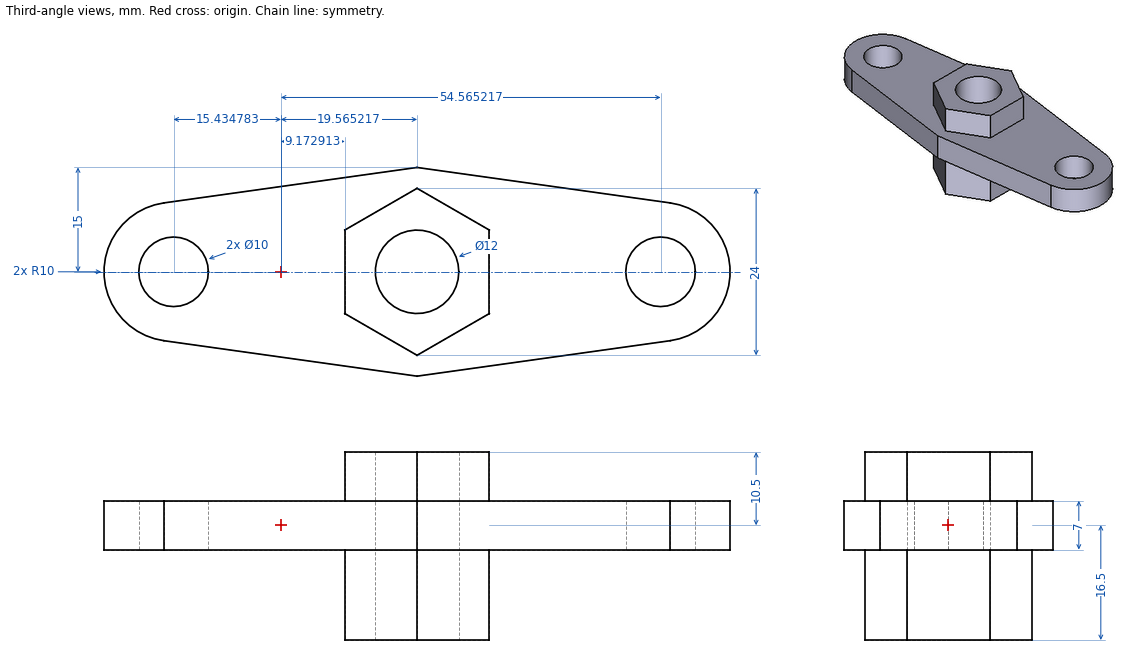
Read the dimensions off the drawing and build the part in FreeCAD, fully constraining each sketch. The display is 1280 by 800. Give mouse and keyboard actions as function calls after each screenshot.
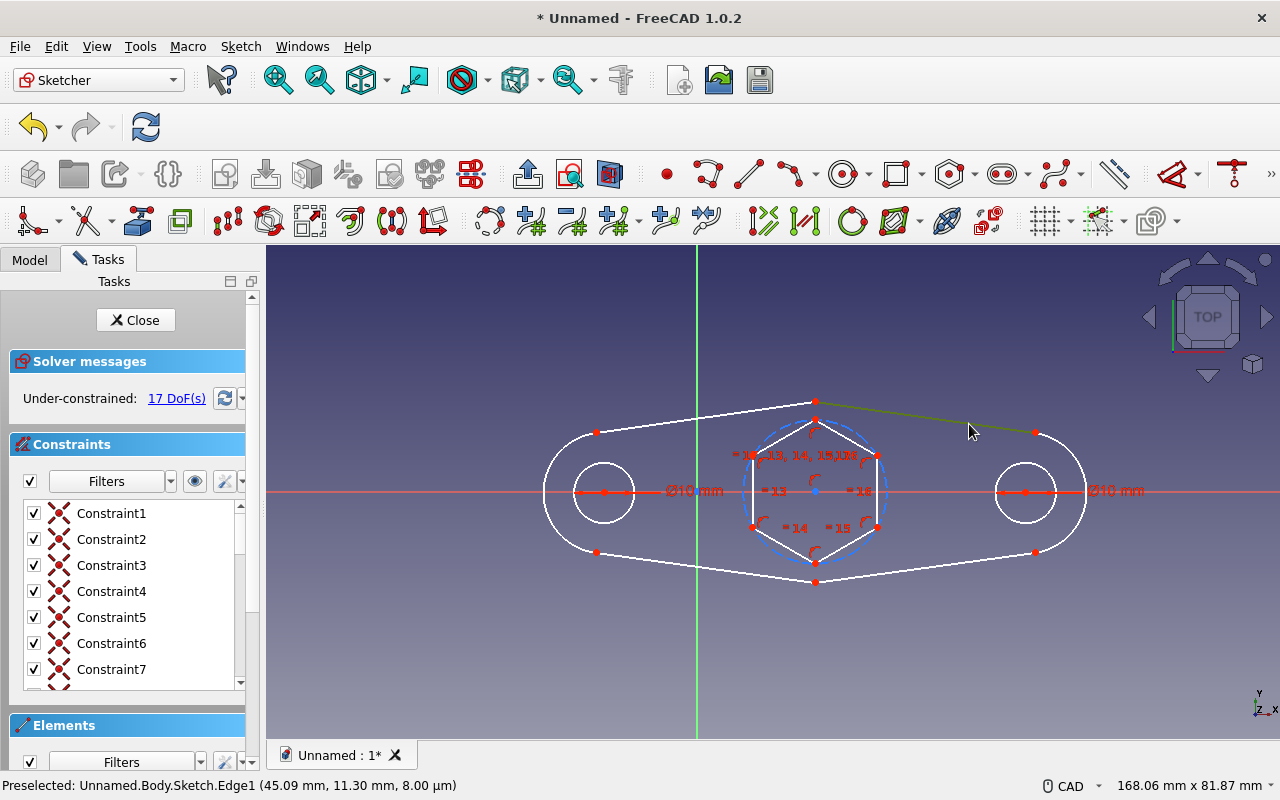
click(1077, 526)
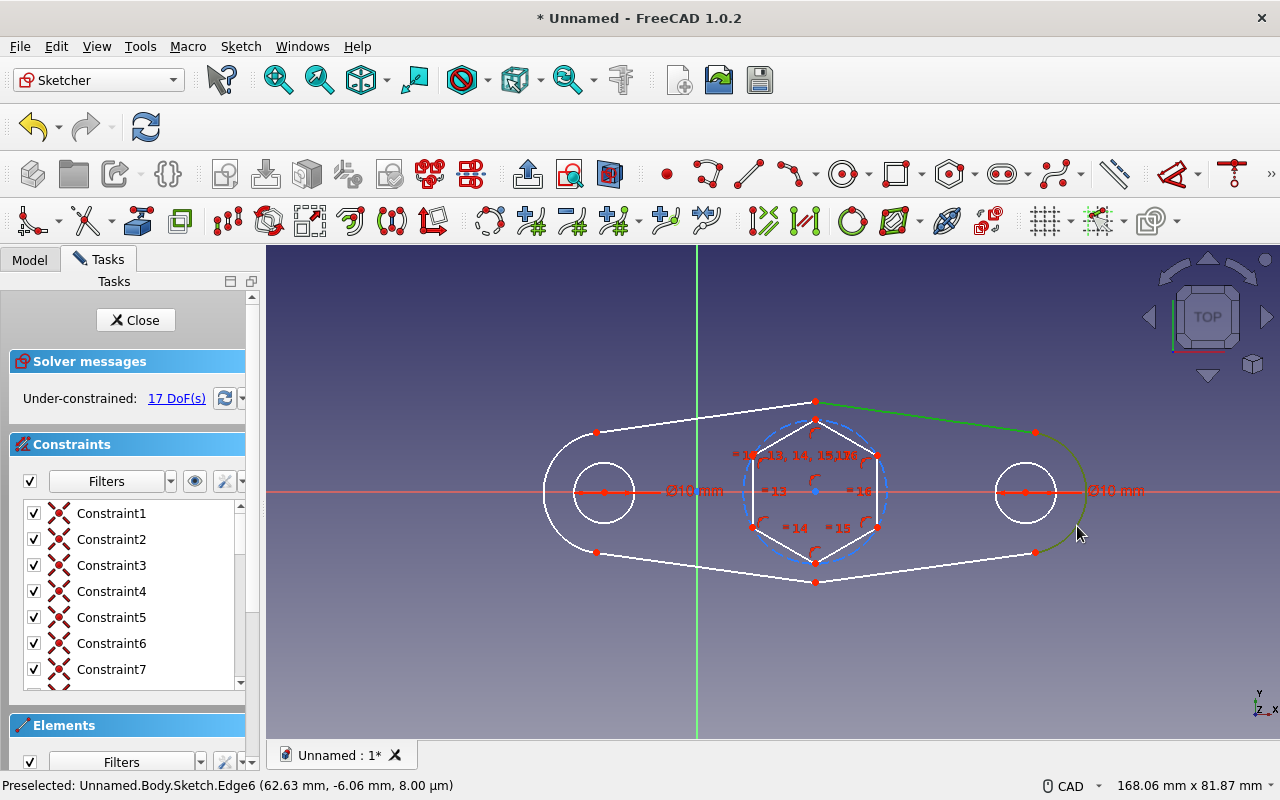
key(t)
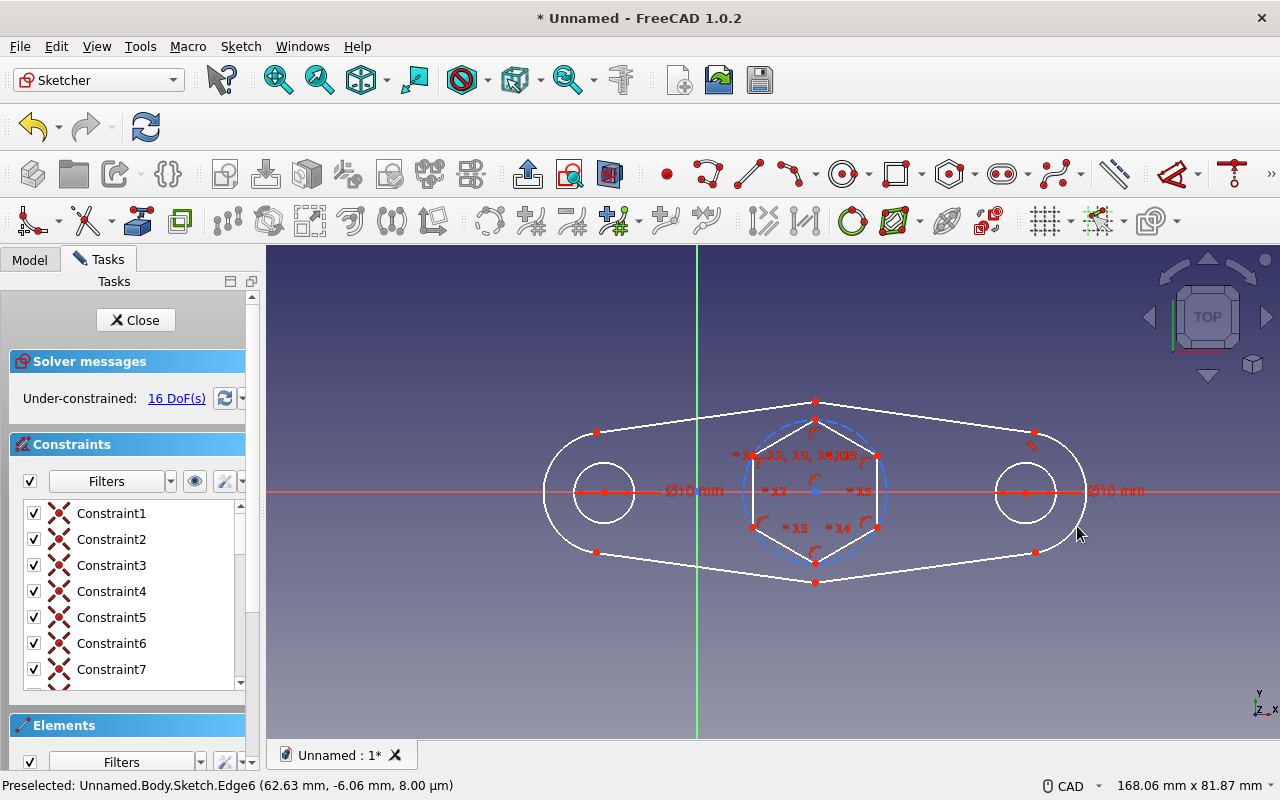
click(749, 411)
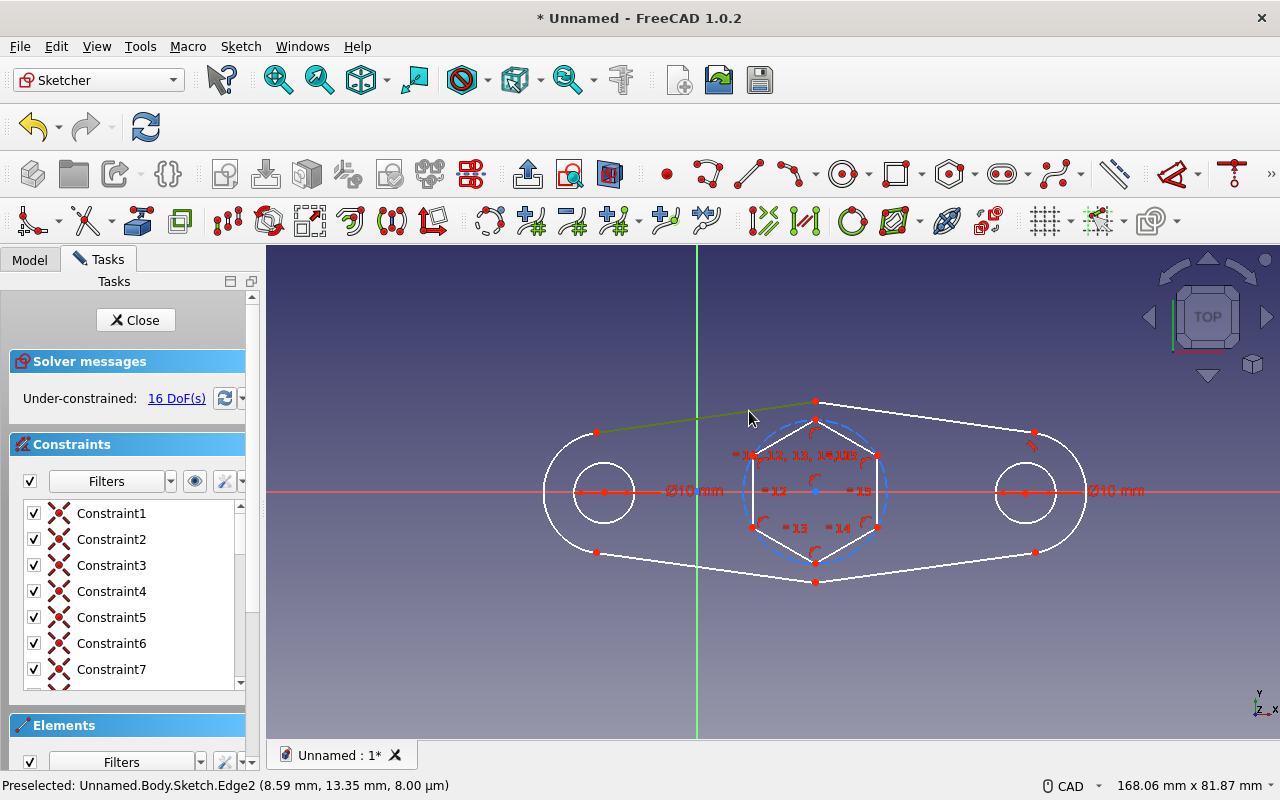
click(553, 460)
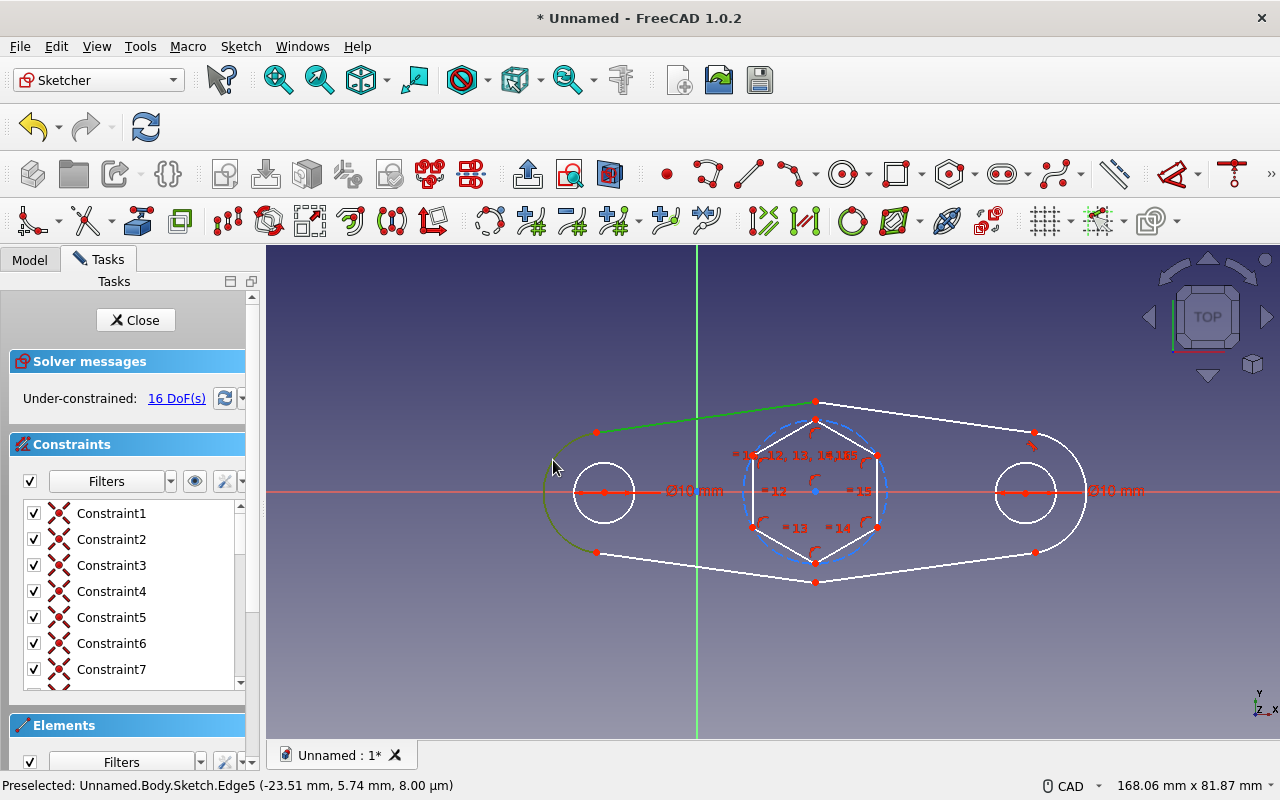
key(t)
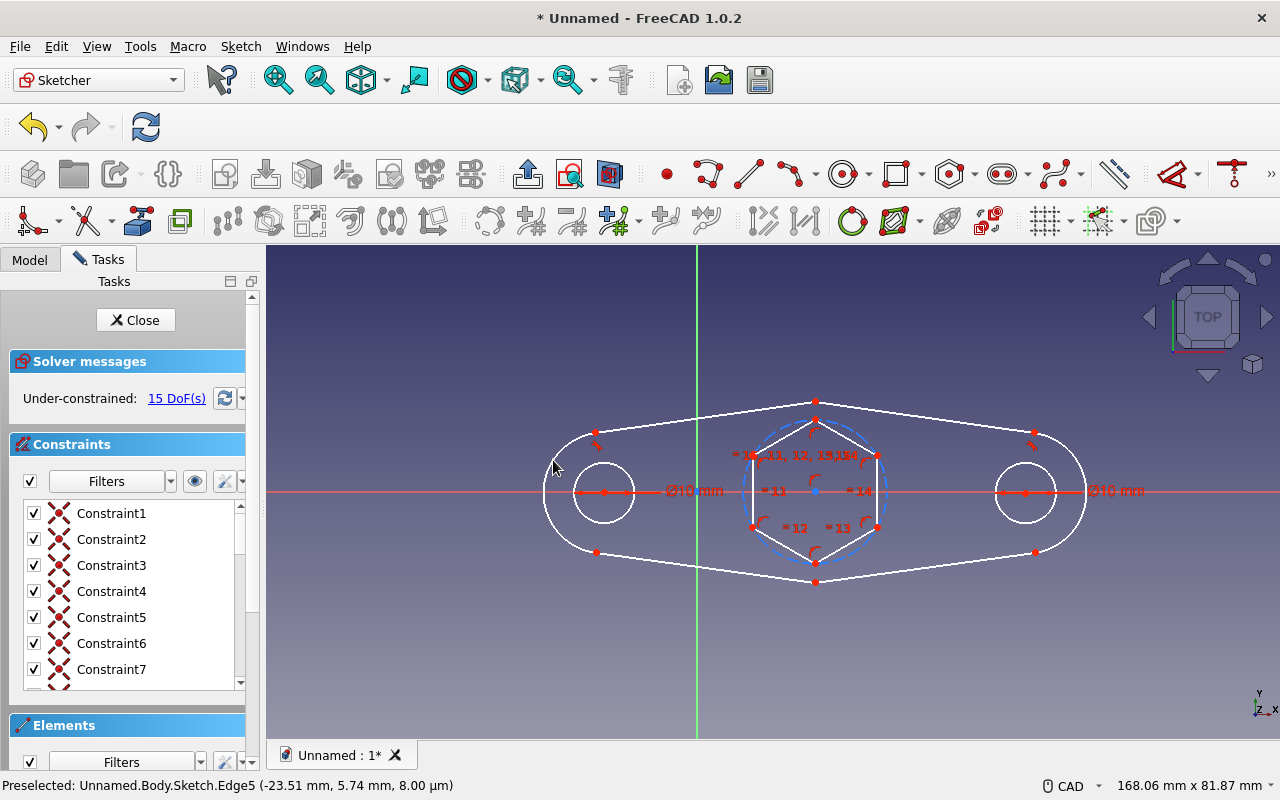
click(662, 562)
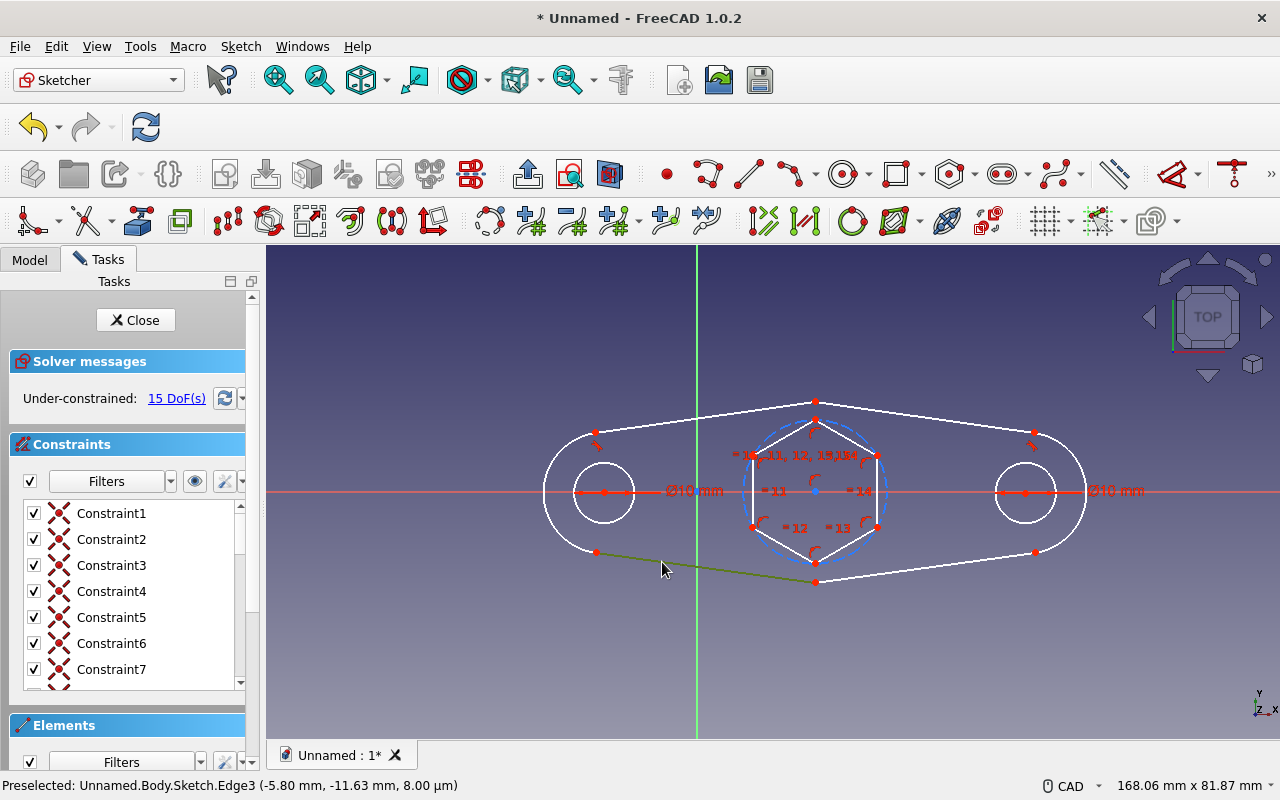
click(553, 460)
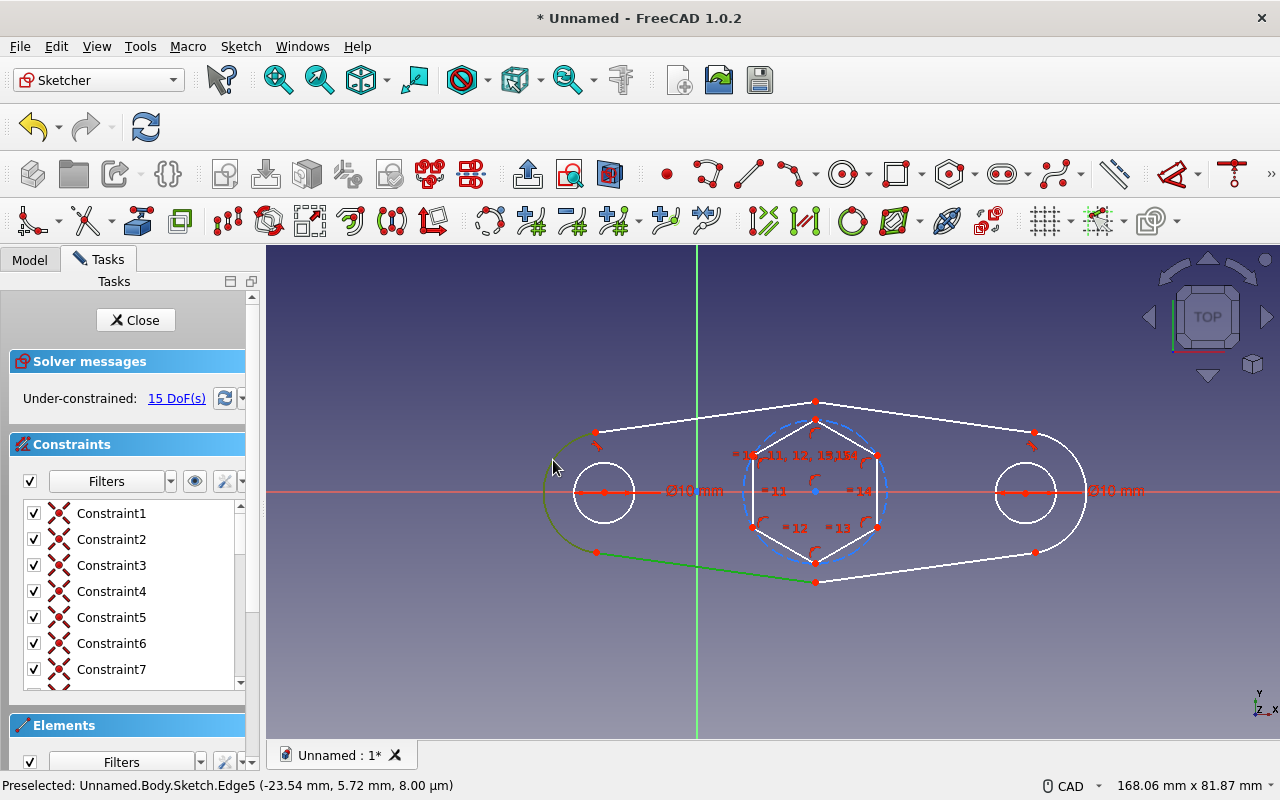
key(t)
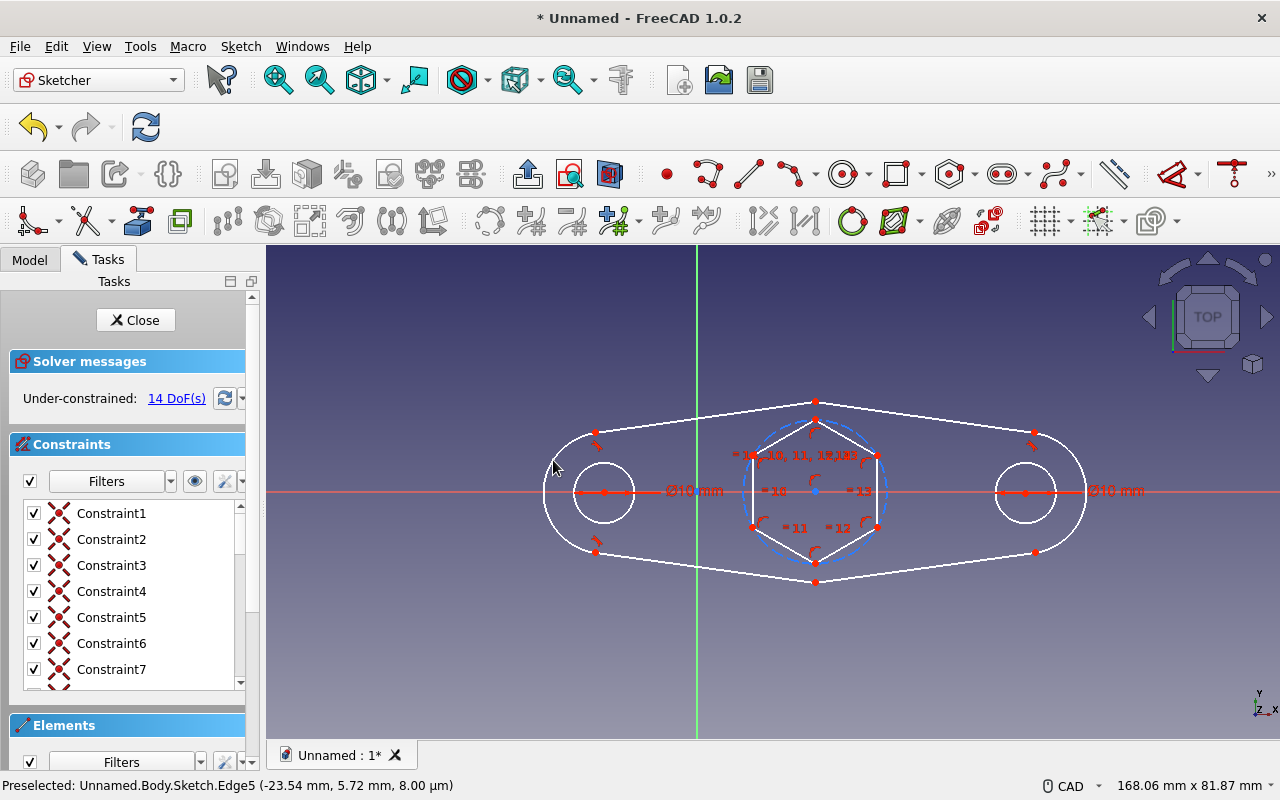
click(881, 574)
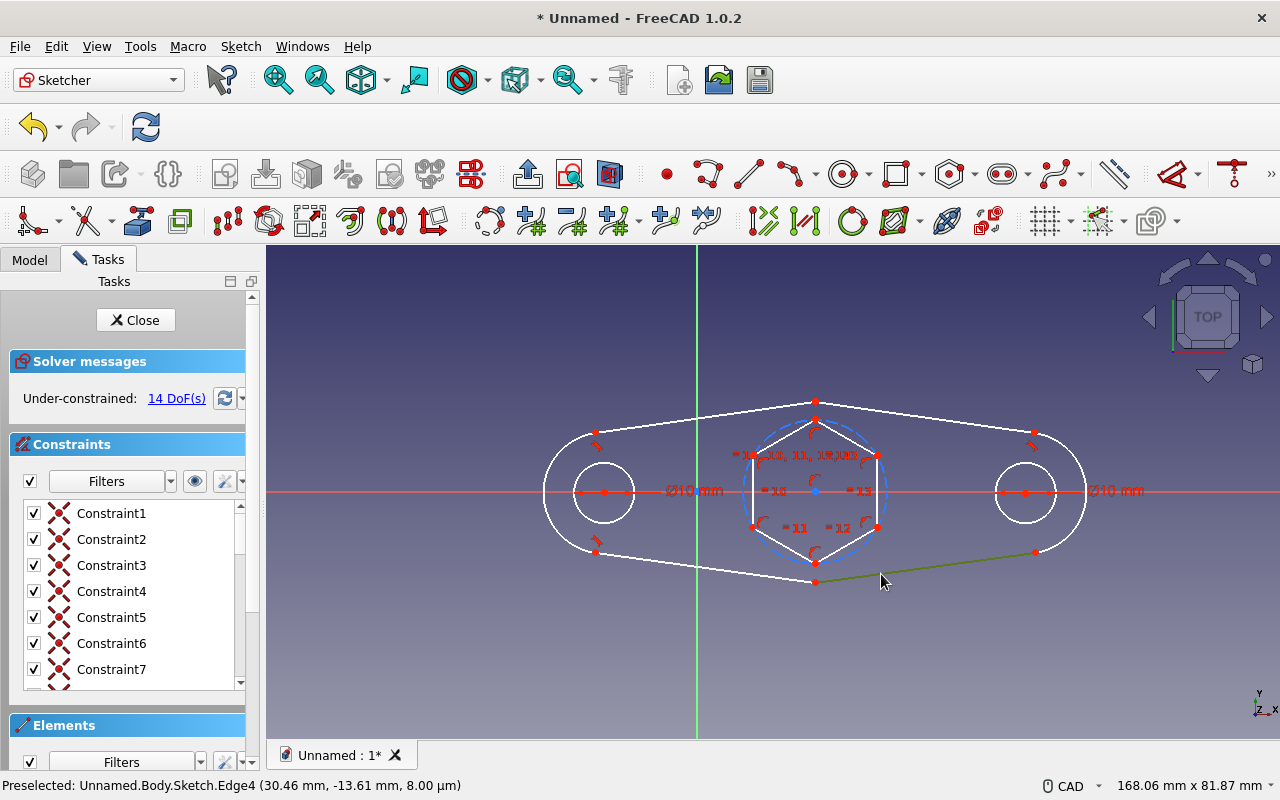
click(1077, 525)